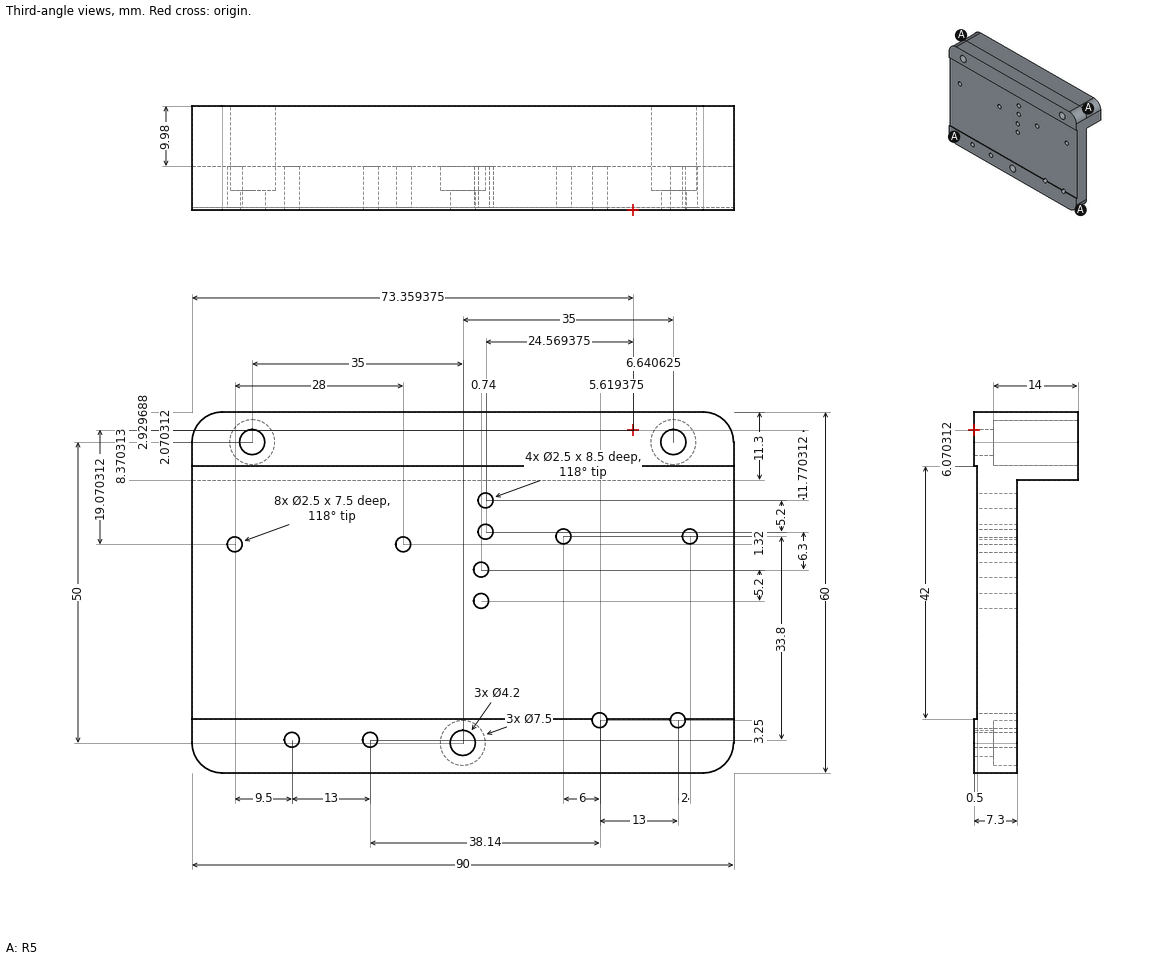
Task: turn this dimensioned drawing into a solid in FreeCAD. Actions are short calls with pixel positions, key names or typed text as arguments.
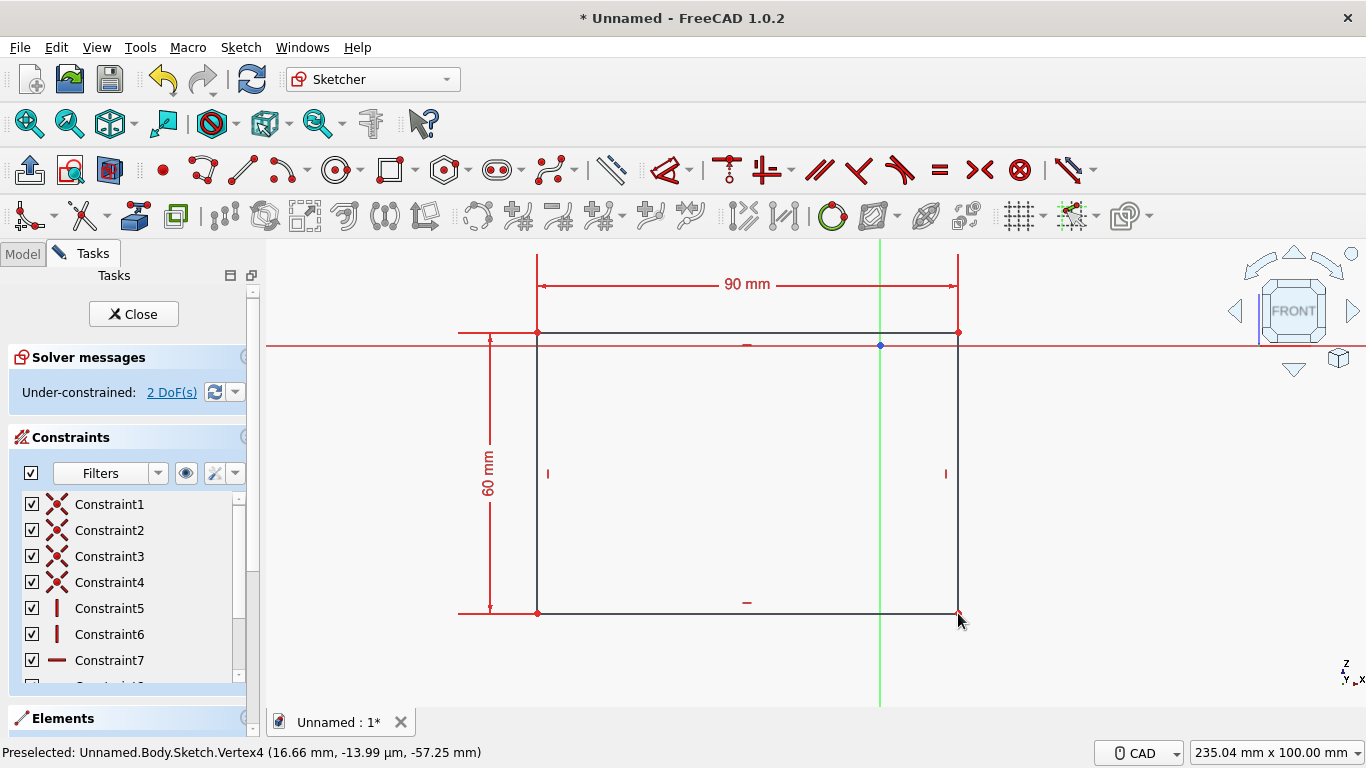
click(666, 170)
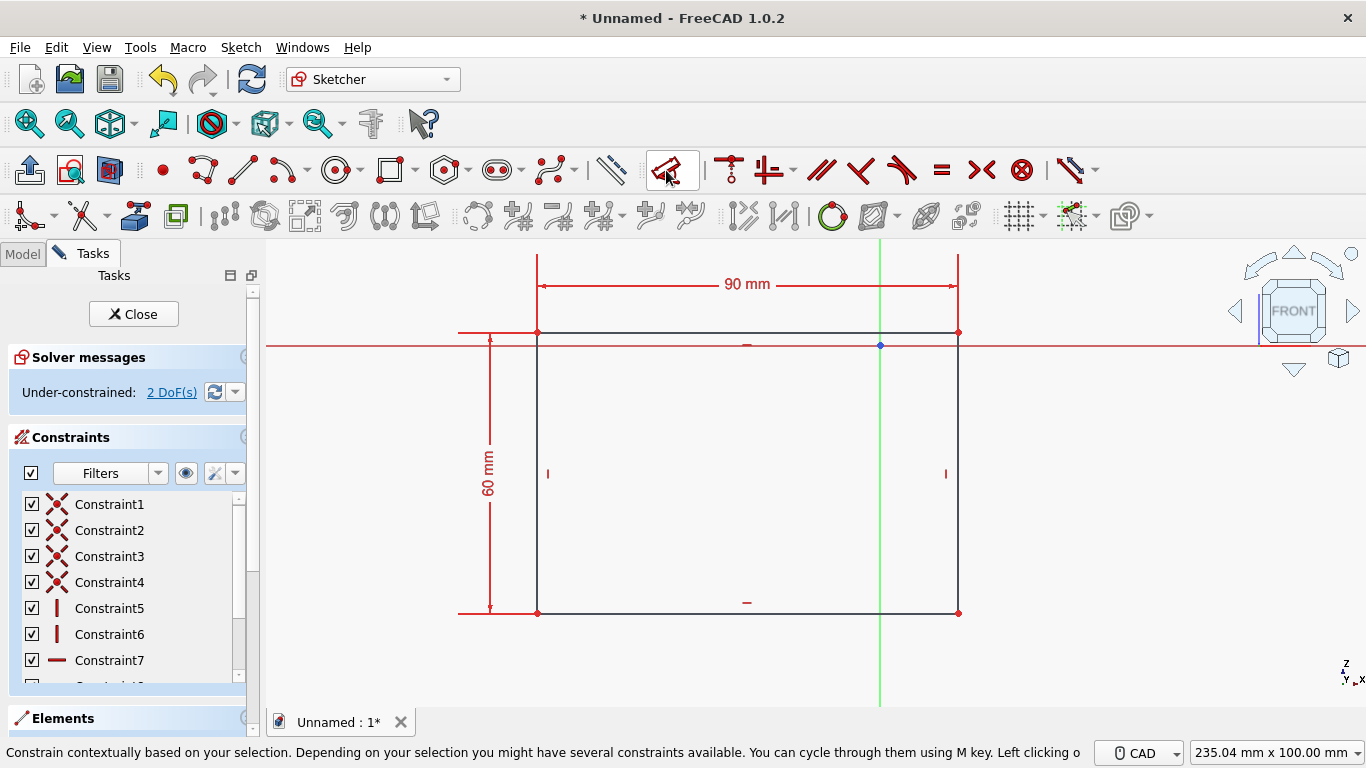
scroll(537, 333, up, 6)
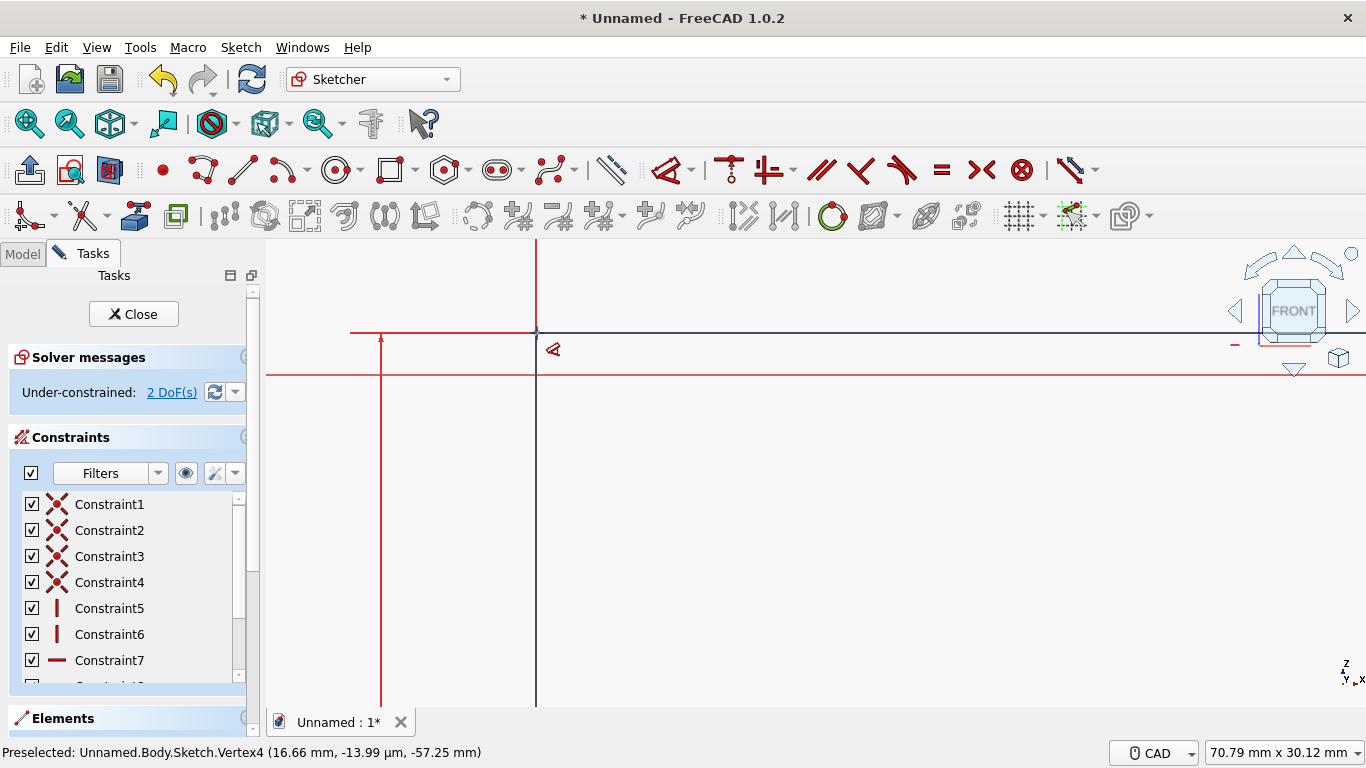
click(536, 333)
click(502, 354)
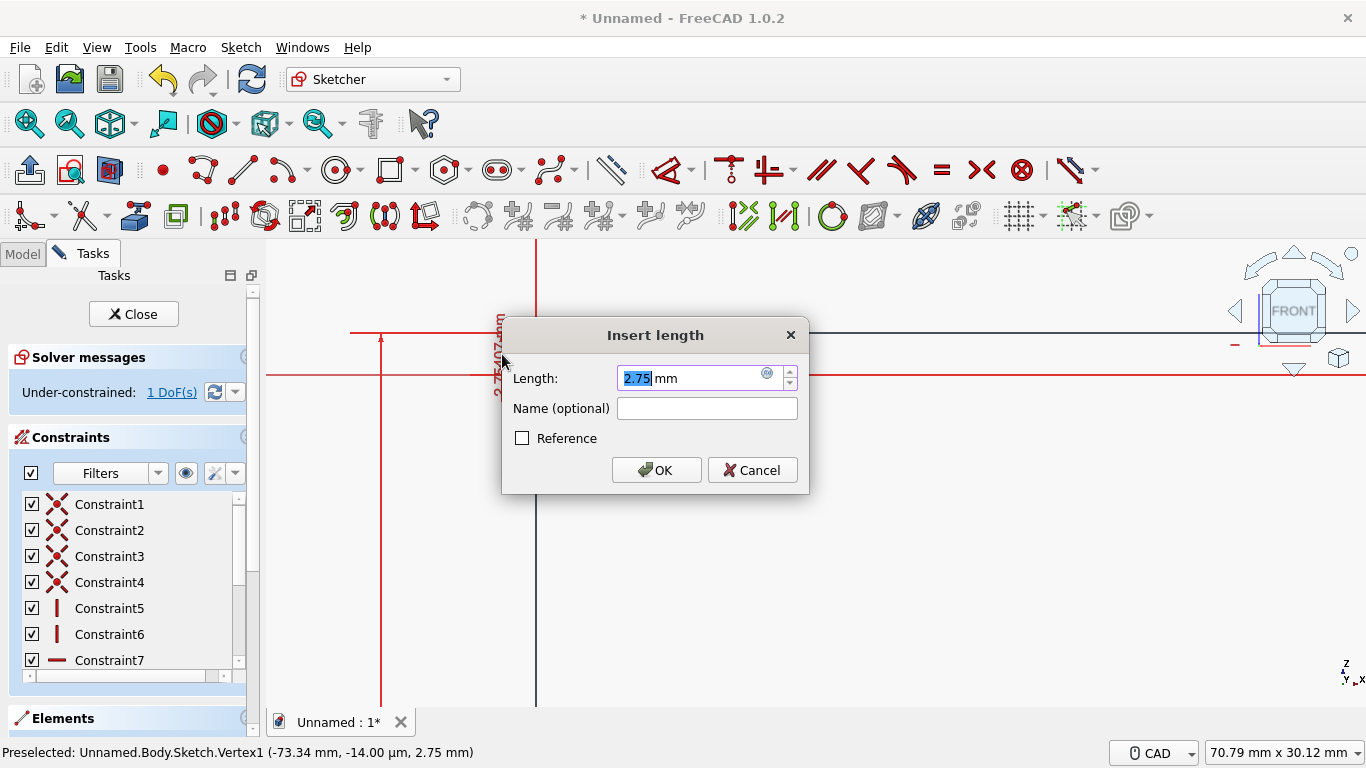
text(2.929688)
key(Return)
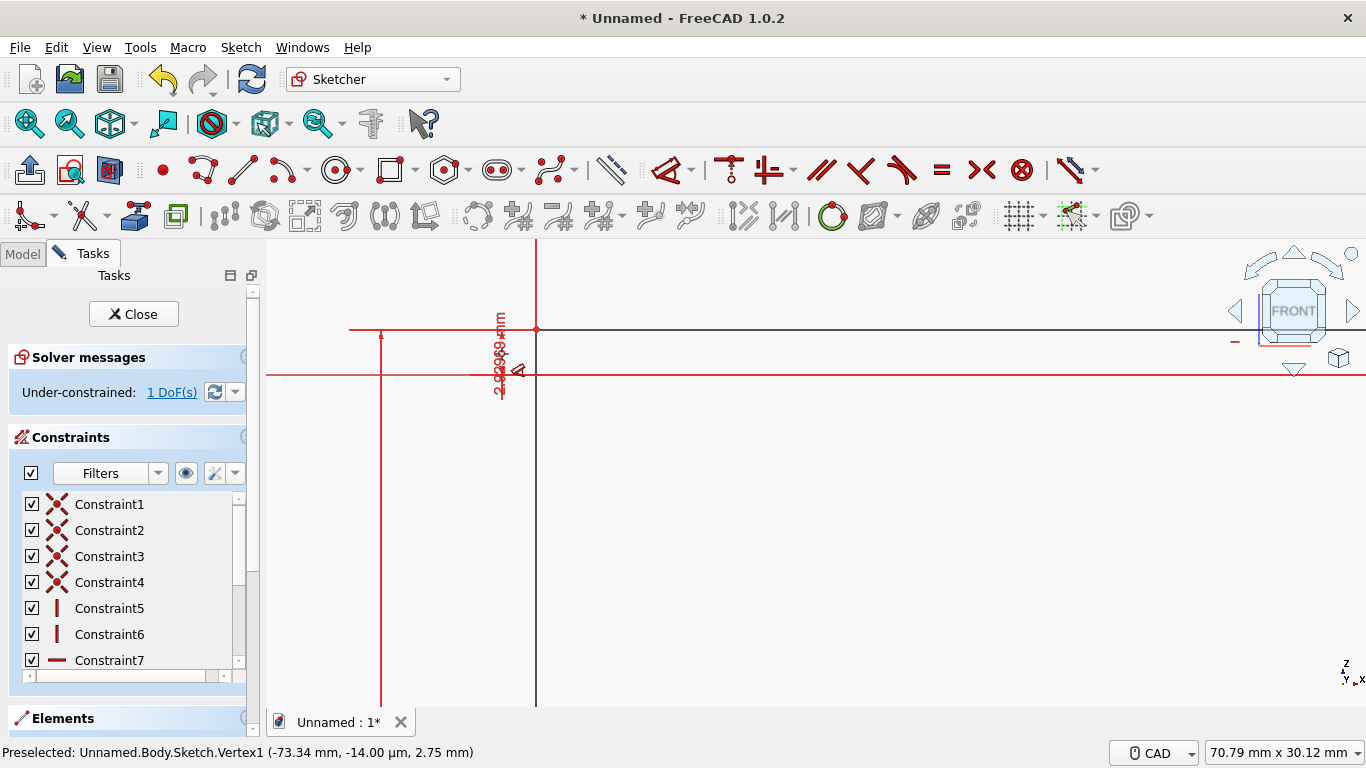
click(536, 330)
click(869, 296)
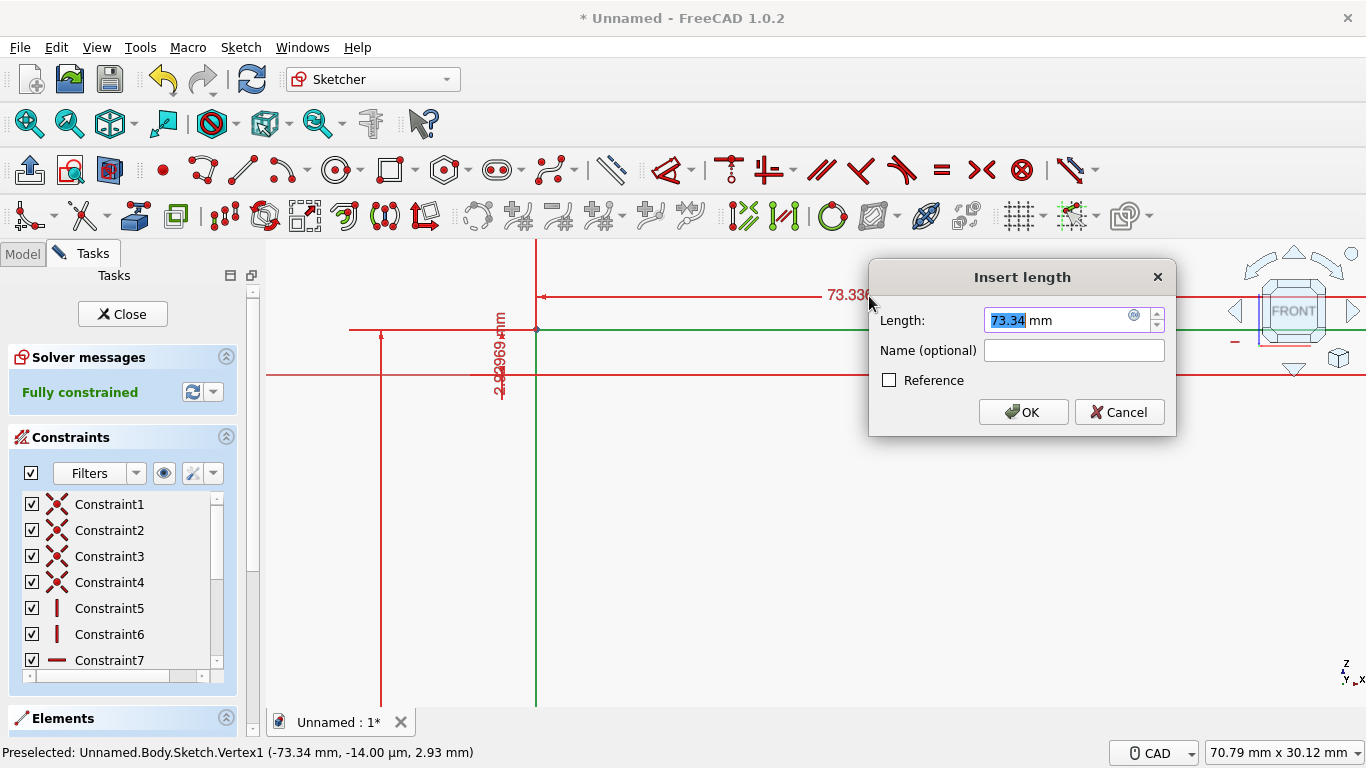
text(73.359375)
key(Return)
key(Escape)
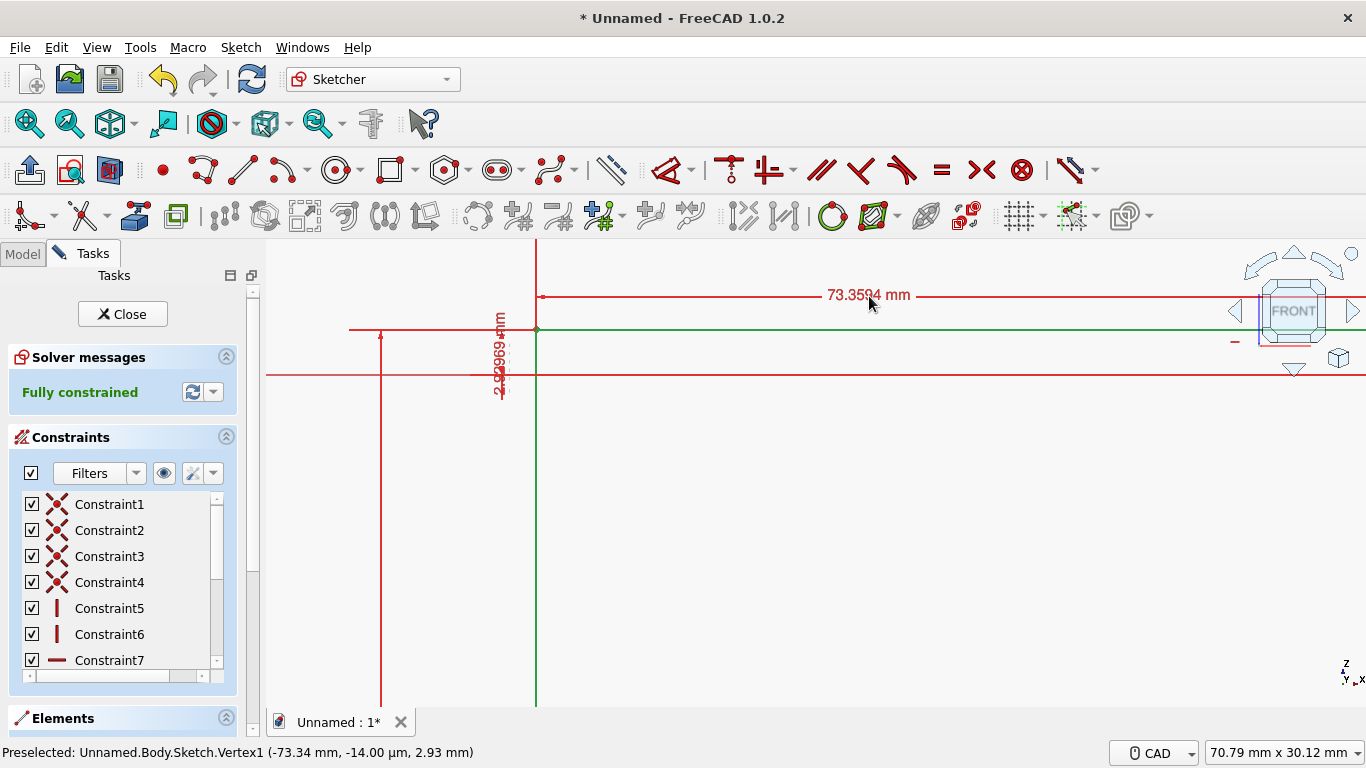
click(123, 314)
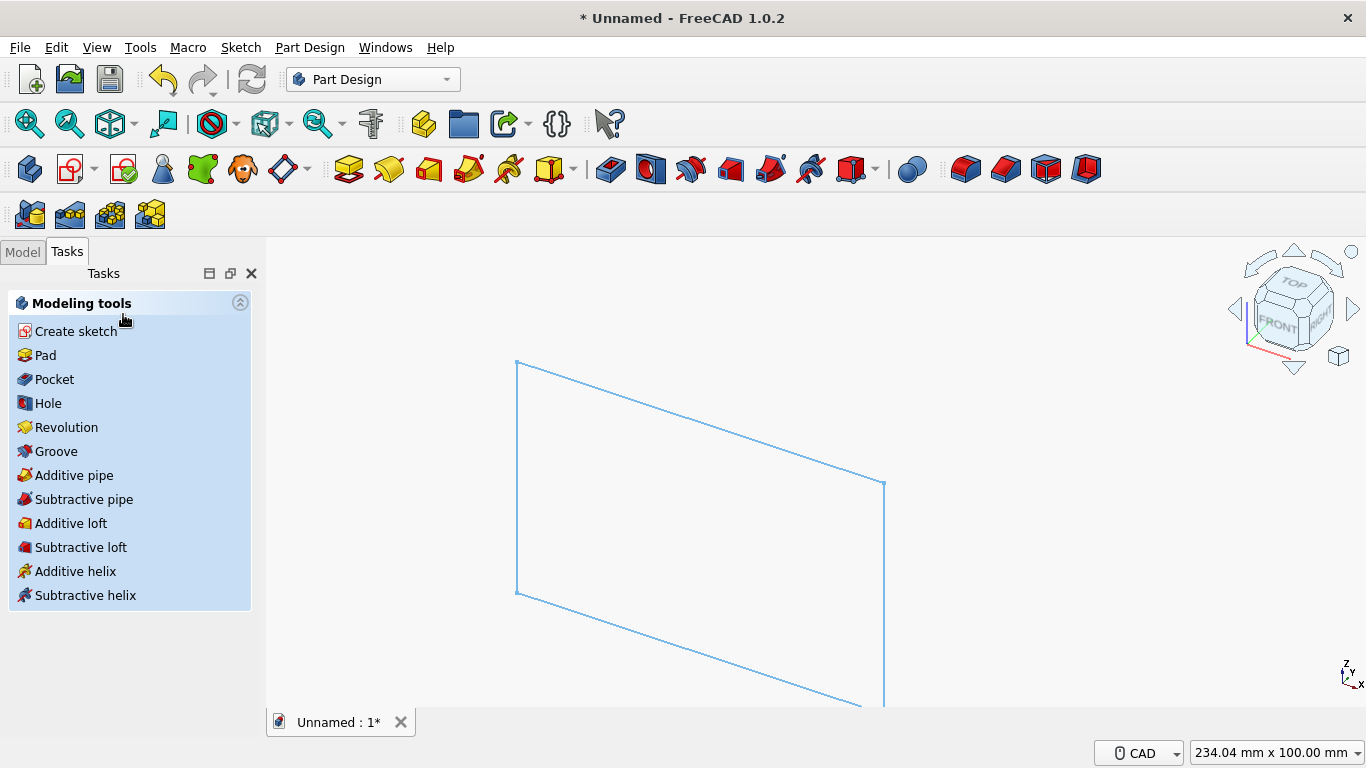
click(350, 170)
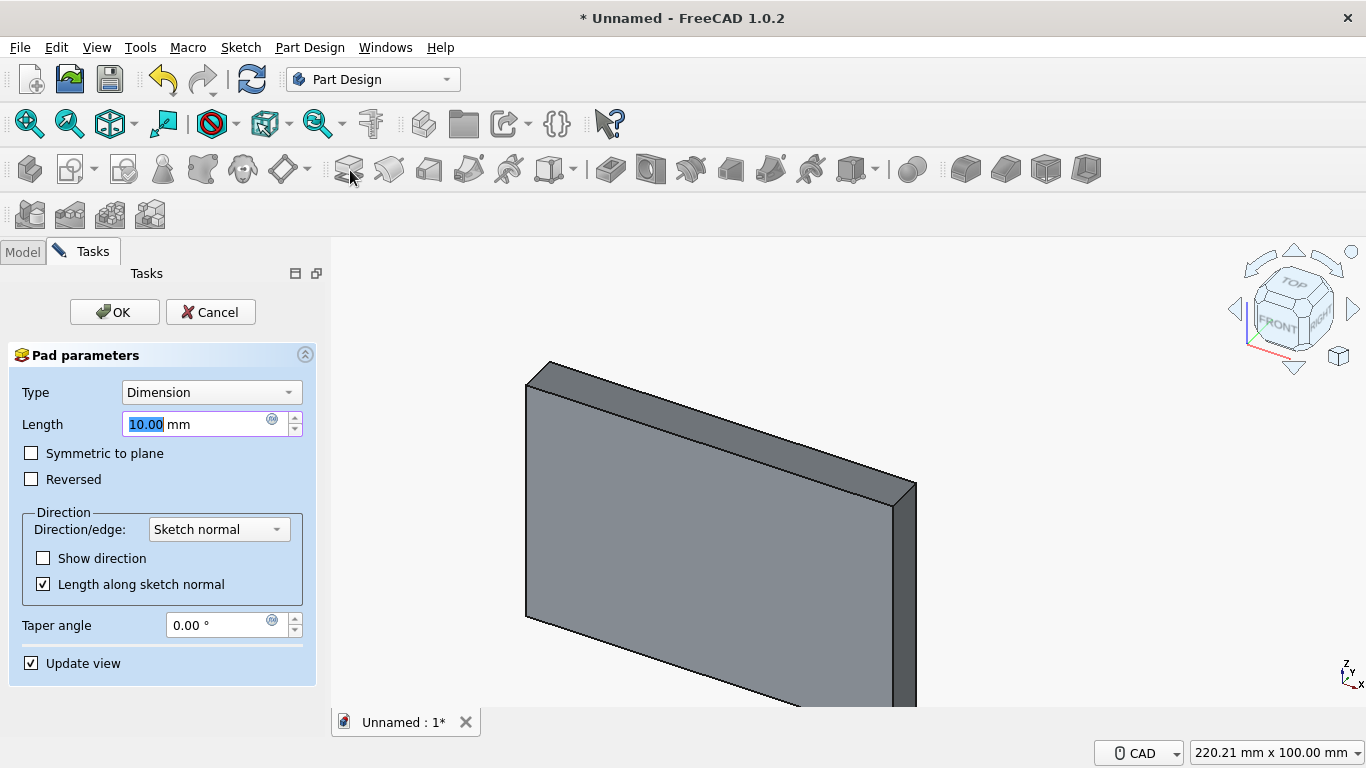
text(7.3)
key(Tab)